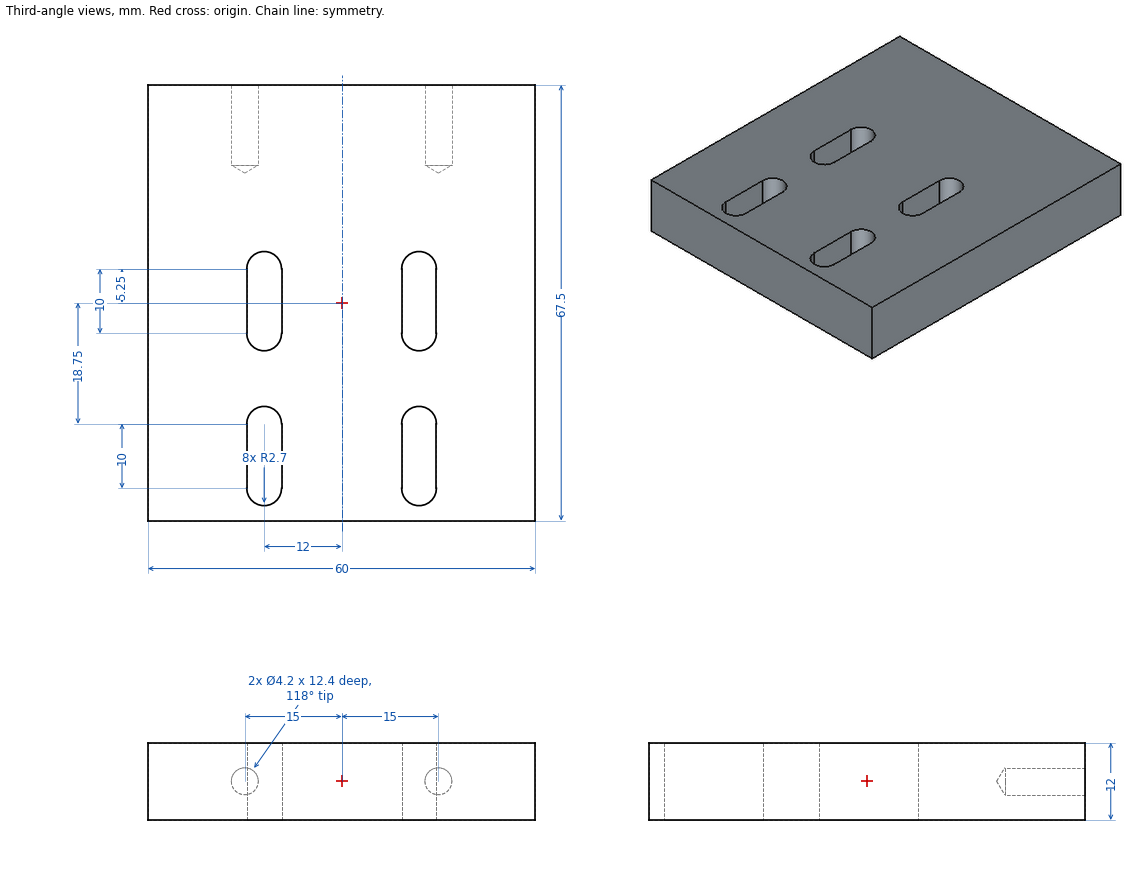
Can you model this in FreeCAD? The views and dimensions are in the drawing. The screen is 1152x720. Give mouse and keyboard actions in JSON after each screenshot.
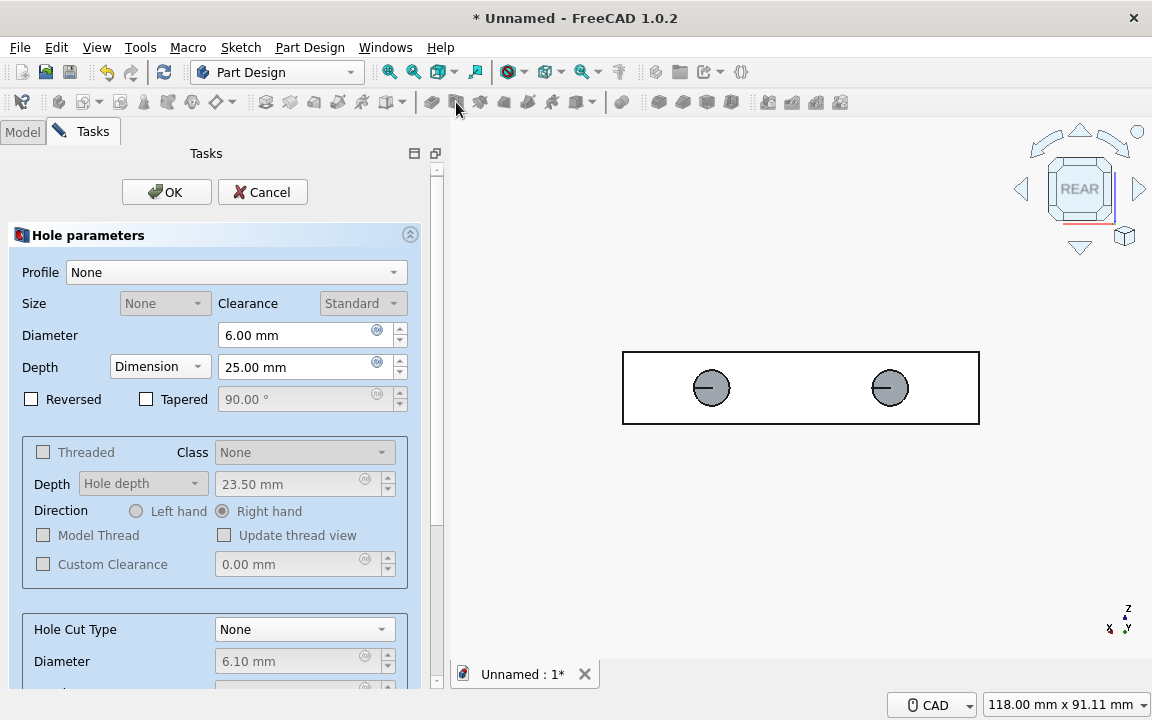
{"action": "triple_click", "coordinate": [305, 335]}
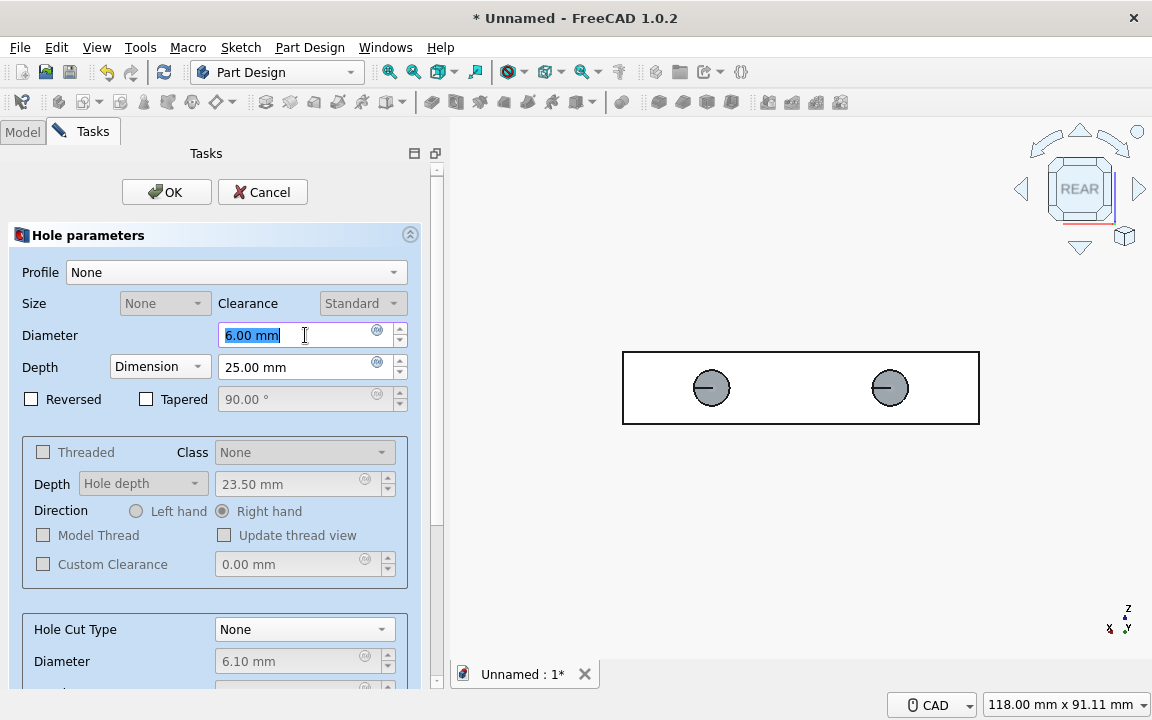
{"action": "type", "text": "4.2"}
{"action": "key", "text": "Tab"}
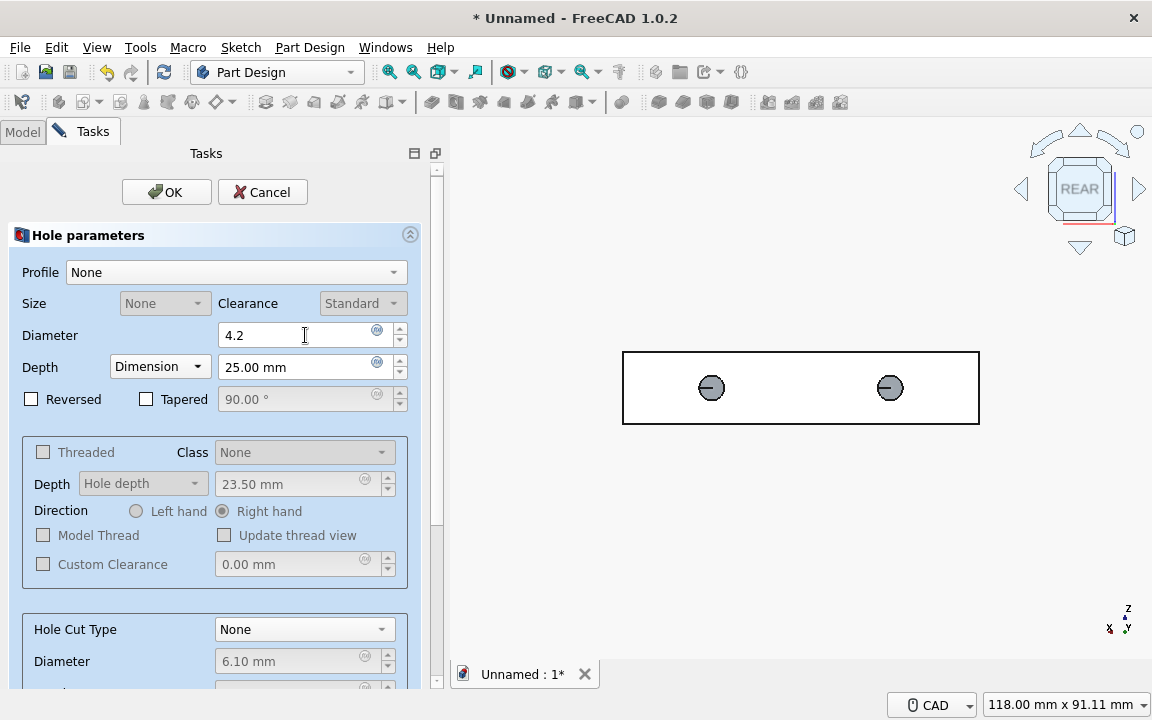
{"action": "triple_click", "coordinate": [305, 367]}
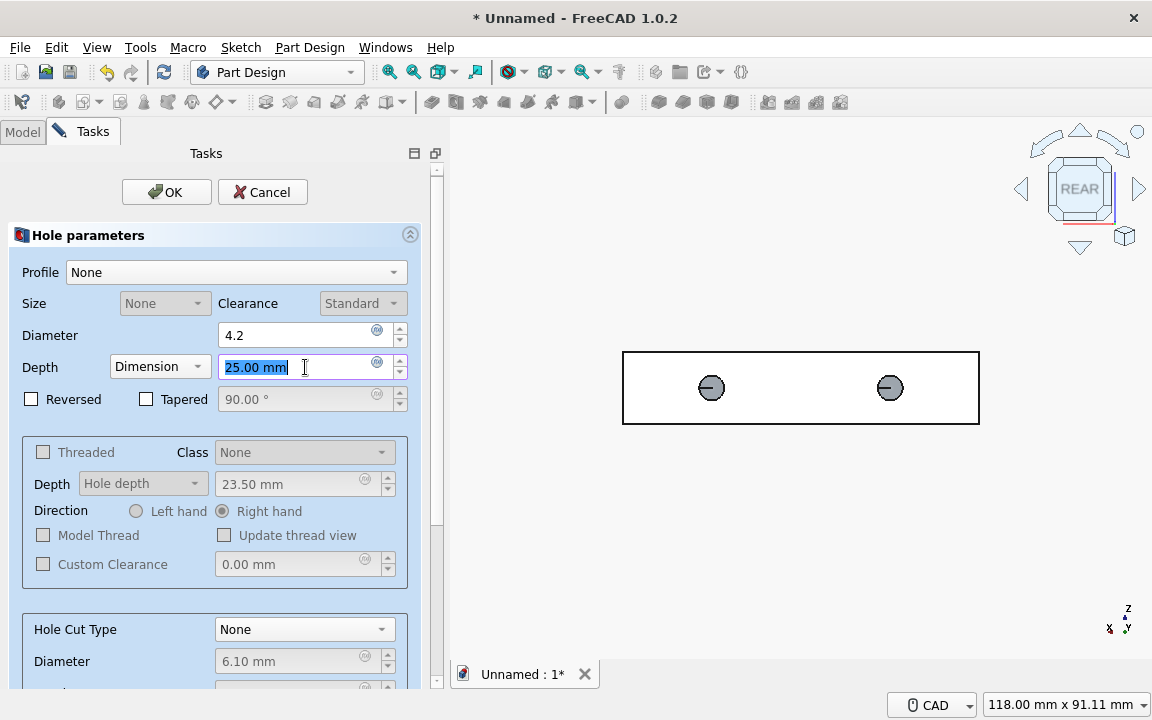
{"action": "type", "text": "12.4"}
{"action": "key", "text": "Tab"}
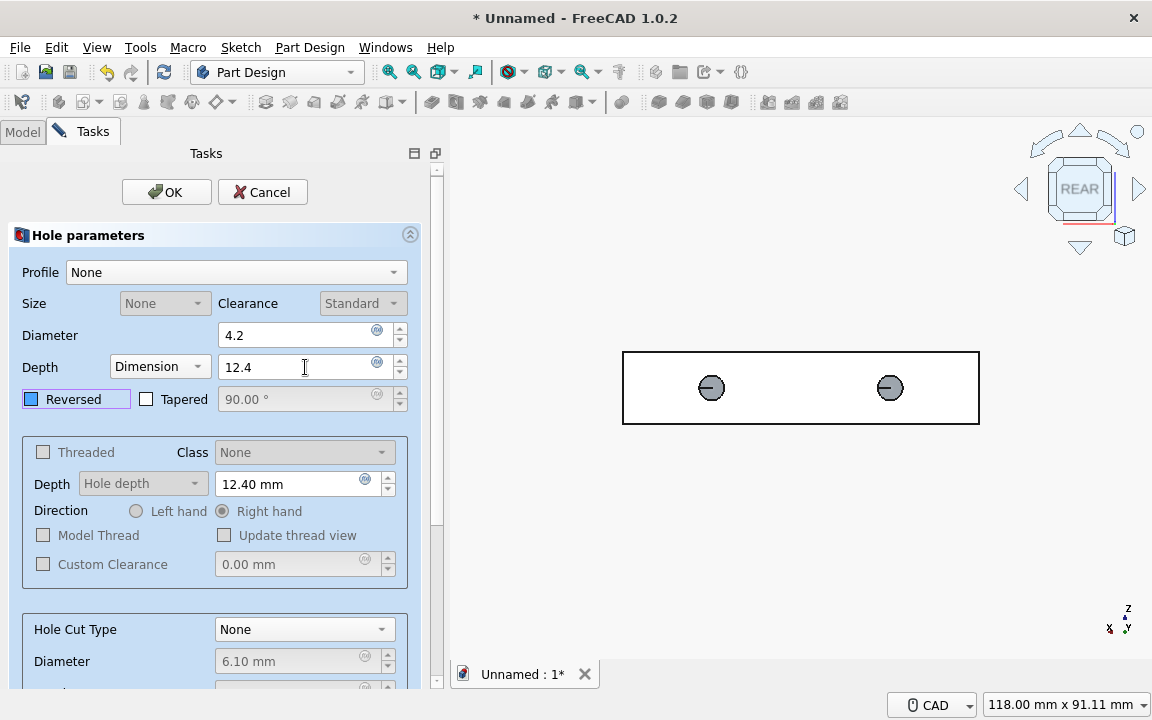
{"action": "left_click", "coordinate": [167, 192]}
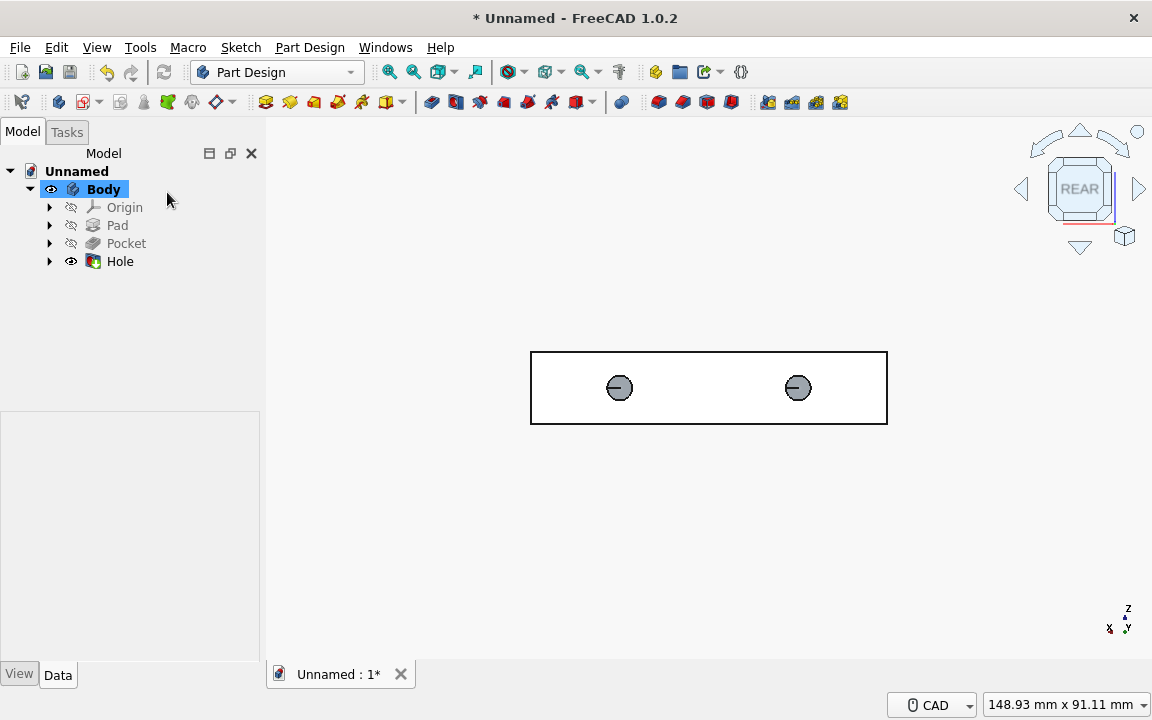
{"action": "key", "text": "0"}